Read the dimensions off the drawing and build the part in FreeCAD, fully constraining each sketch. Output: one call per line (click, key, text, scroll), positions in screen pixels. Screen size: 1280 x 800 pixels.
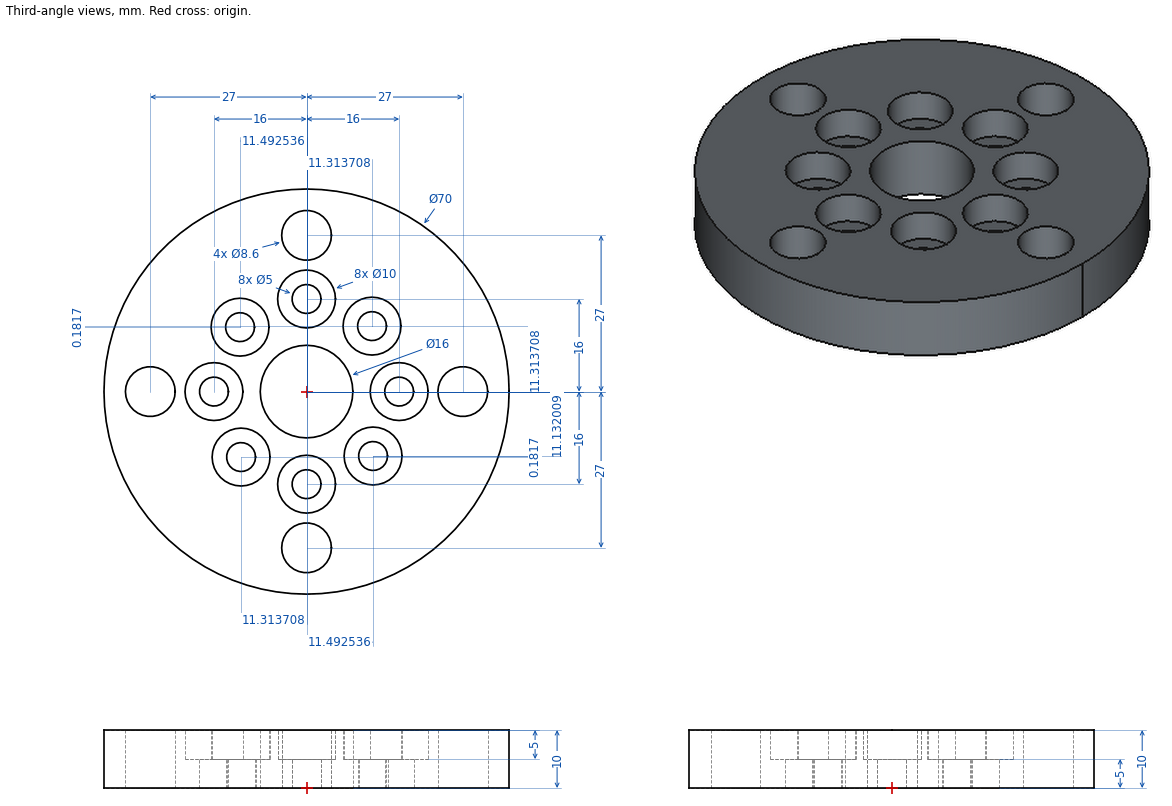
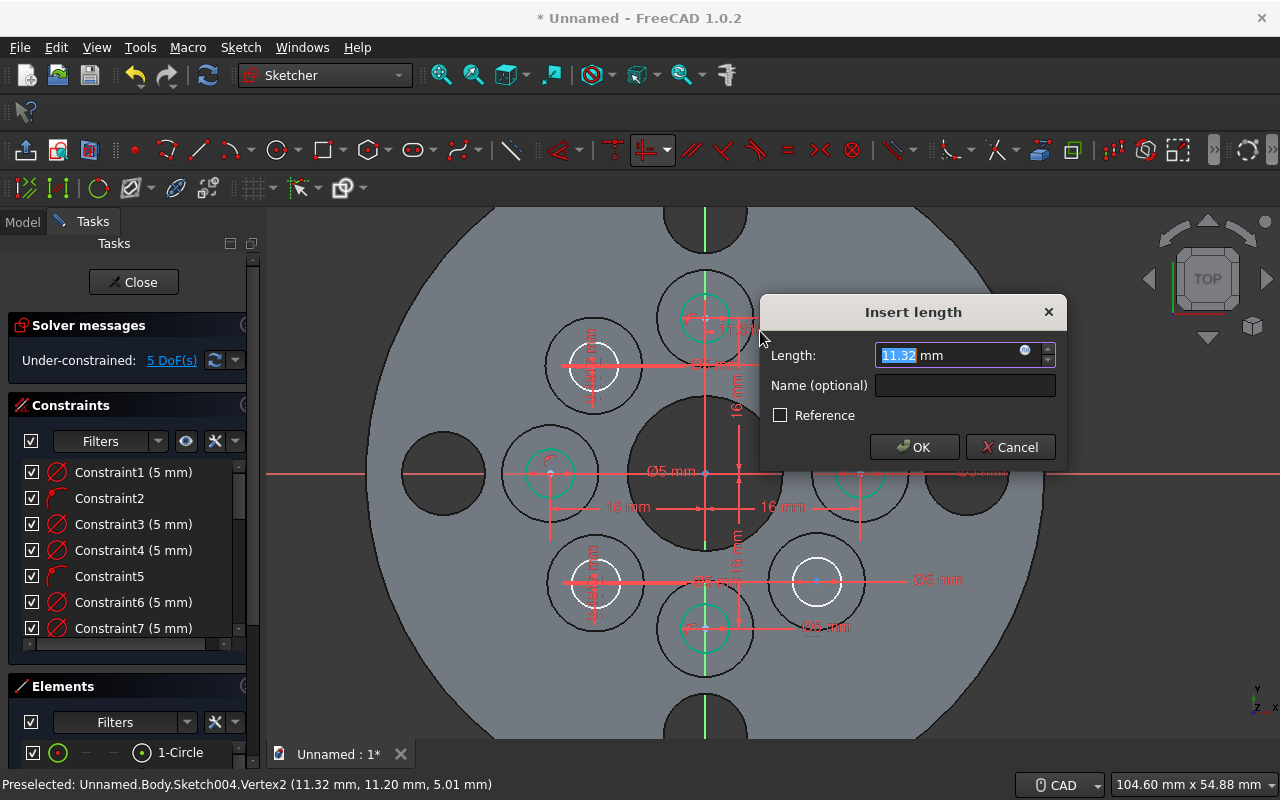
text(11.313708)
key(Return)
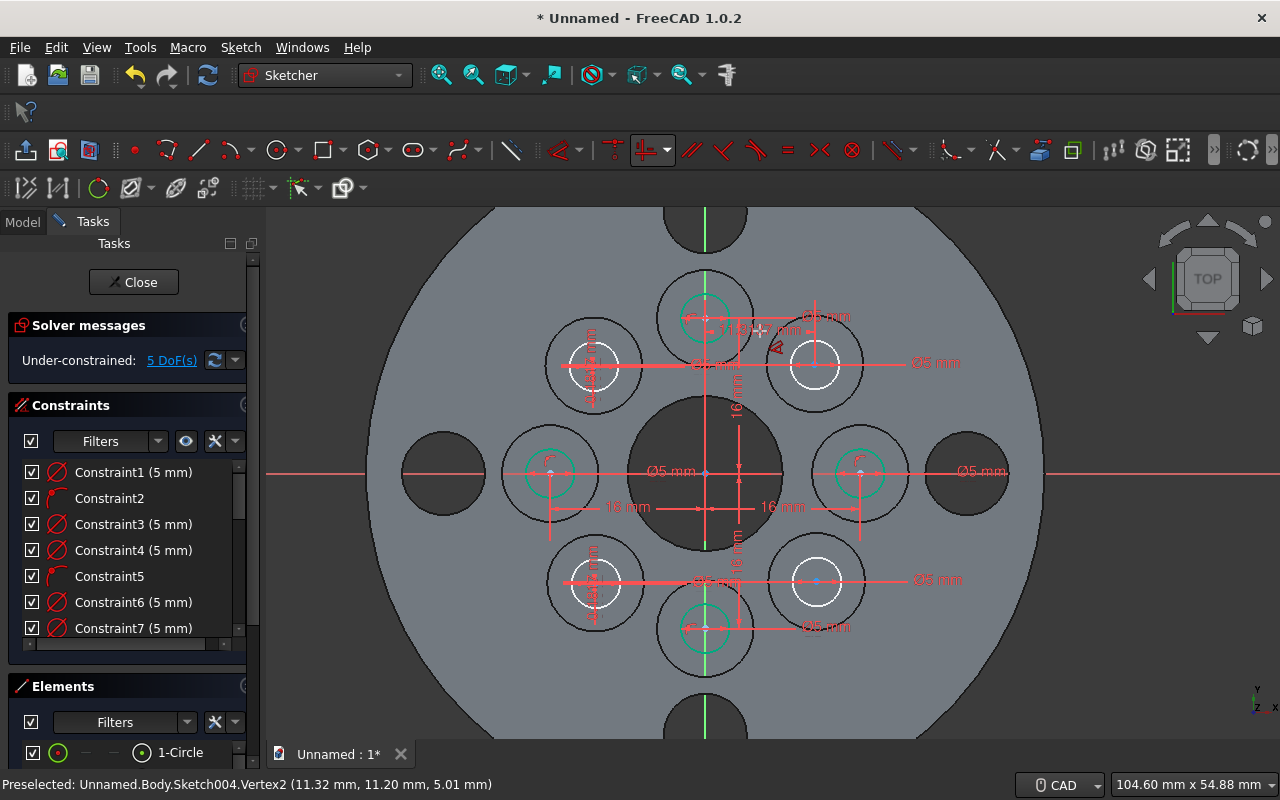
click(815, 365)
click(849, 419)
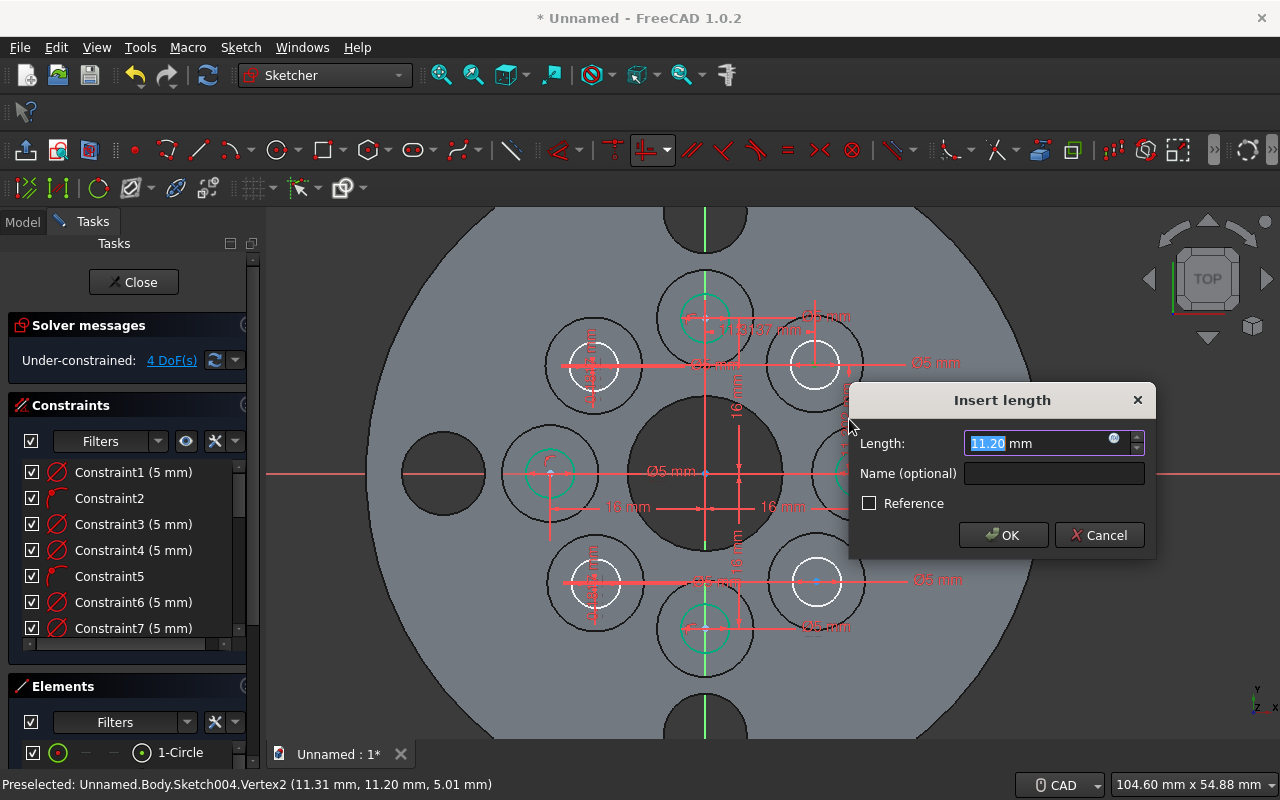
text(11.313708)
key(Return)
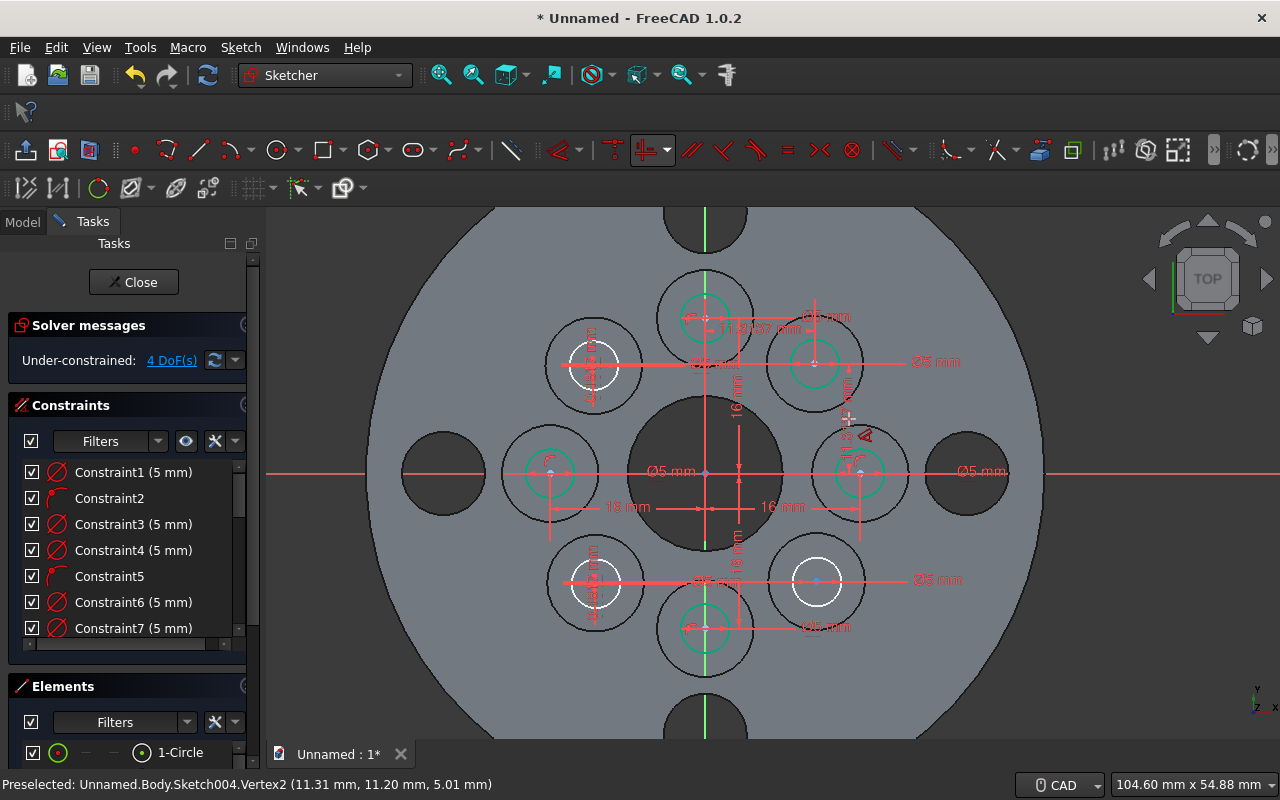
click(817, 582)
click(761, 616)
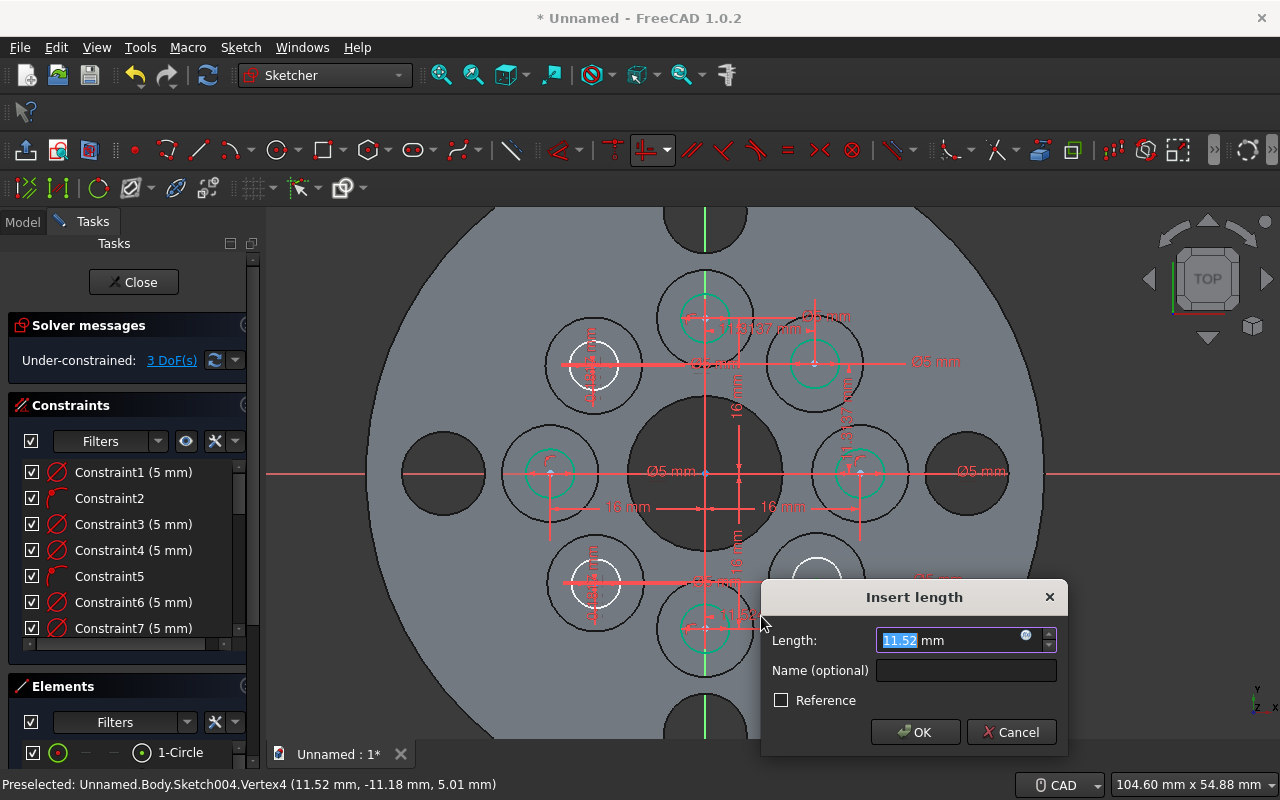
text(11.492536)
key(Return)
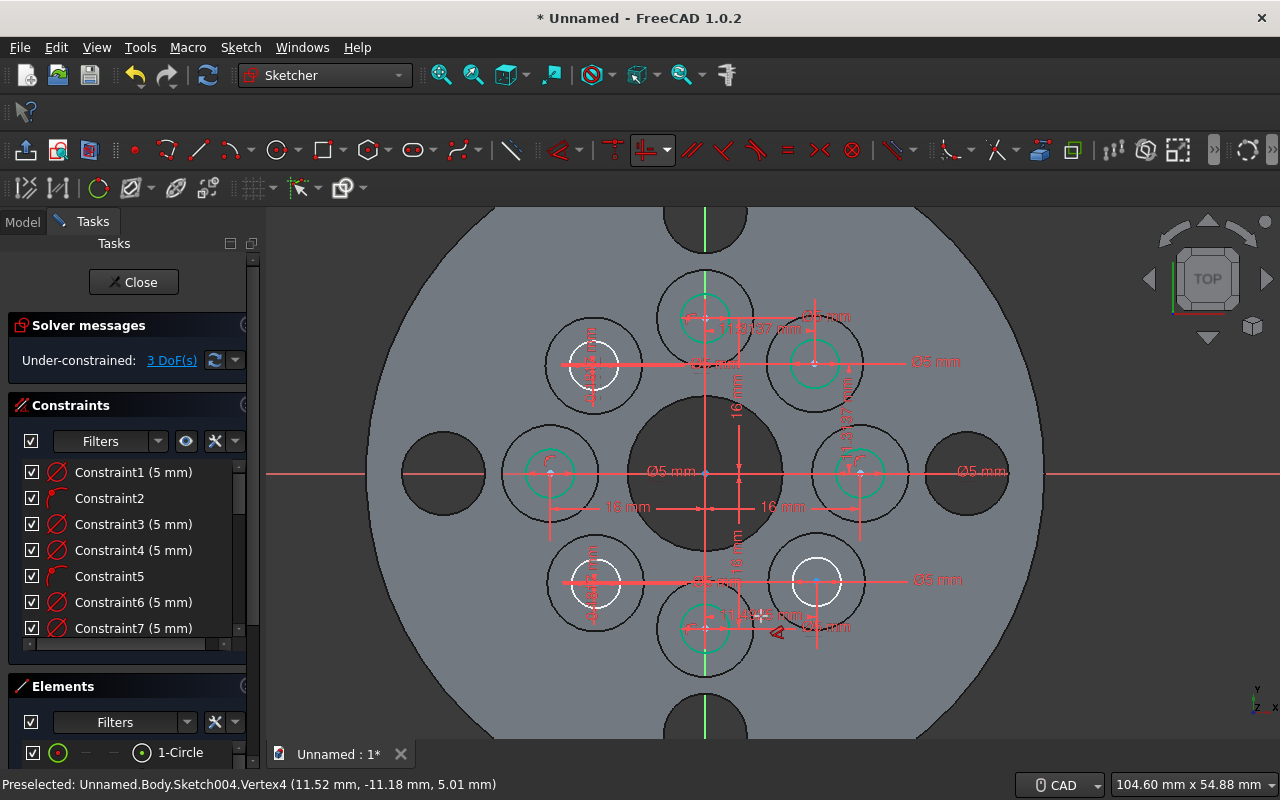
click(817, 582)
click(851, 528)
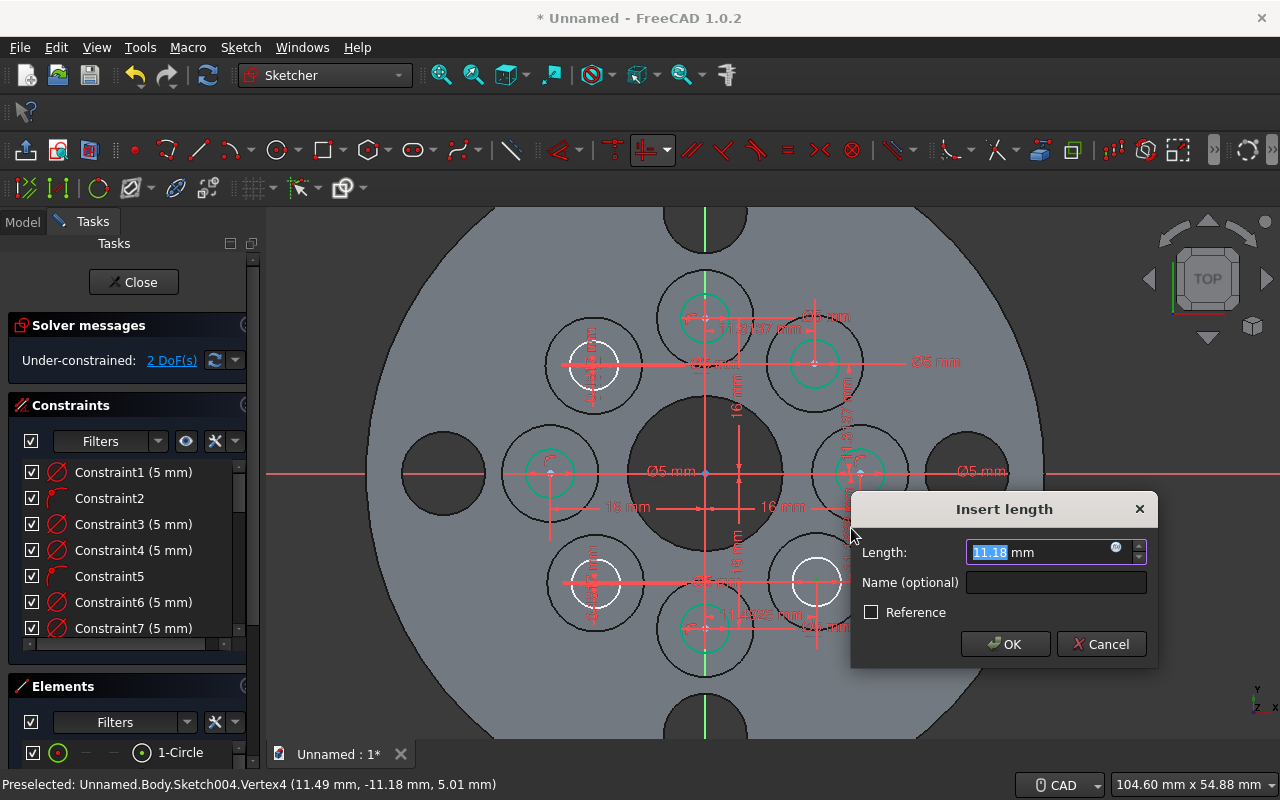
text(11.132009)
key(Return)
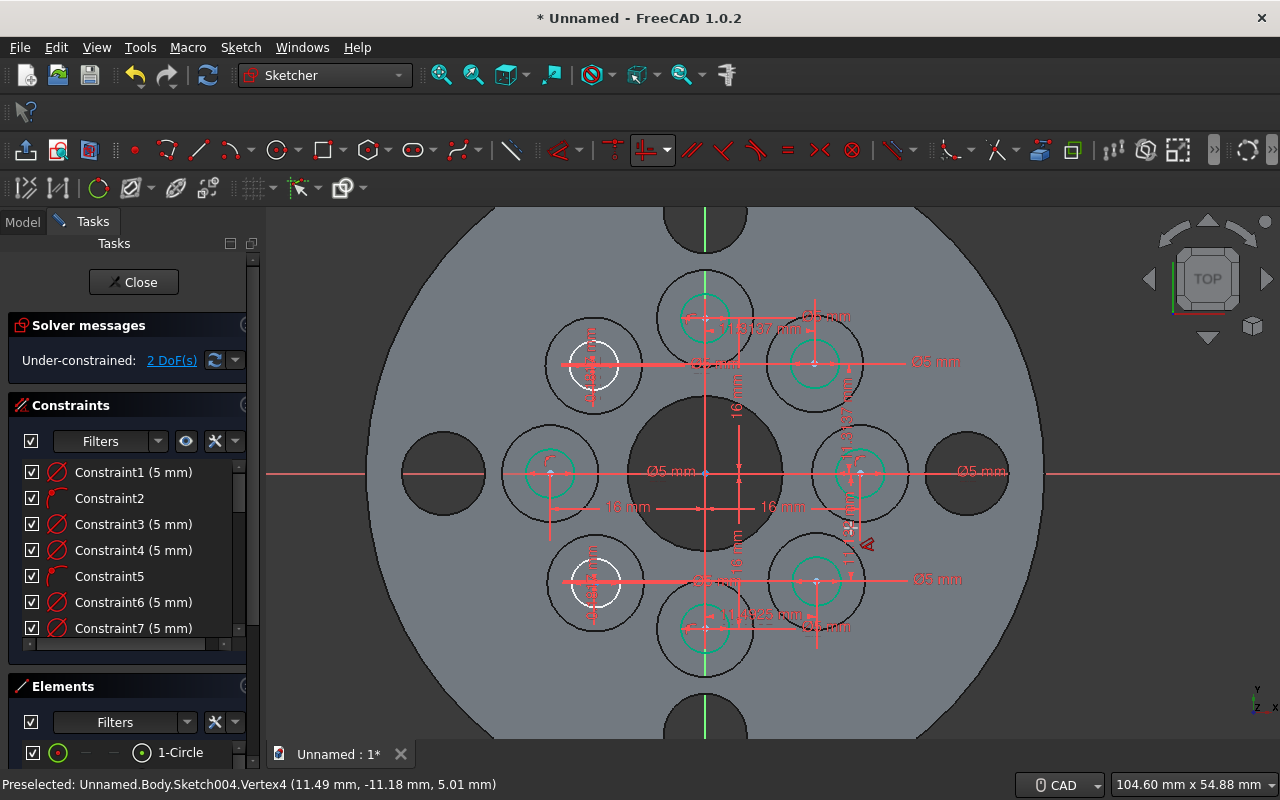
click(596, 583)
click(651, 617)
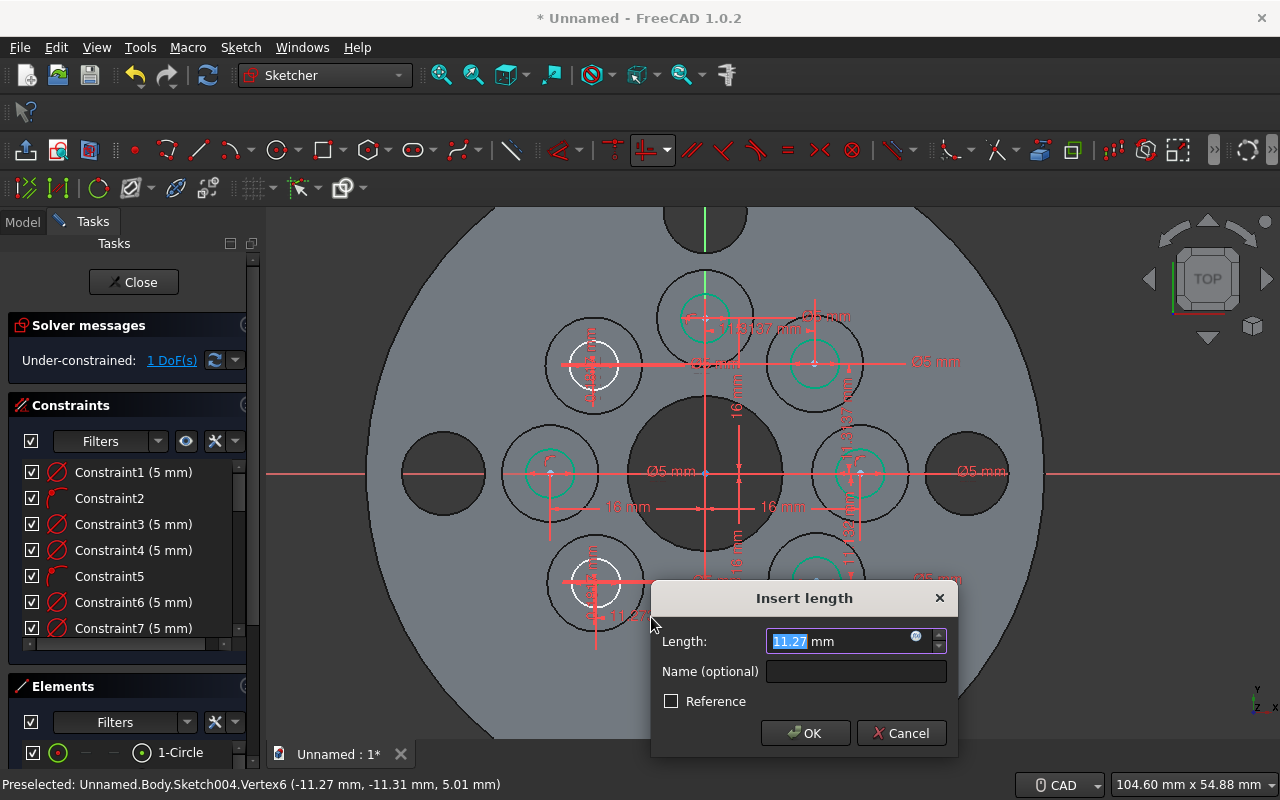
text(11.313708)
key(Return)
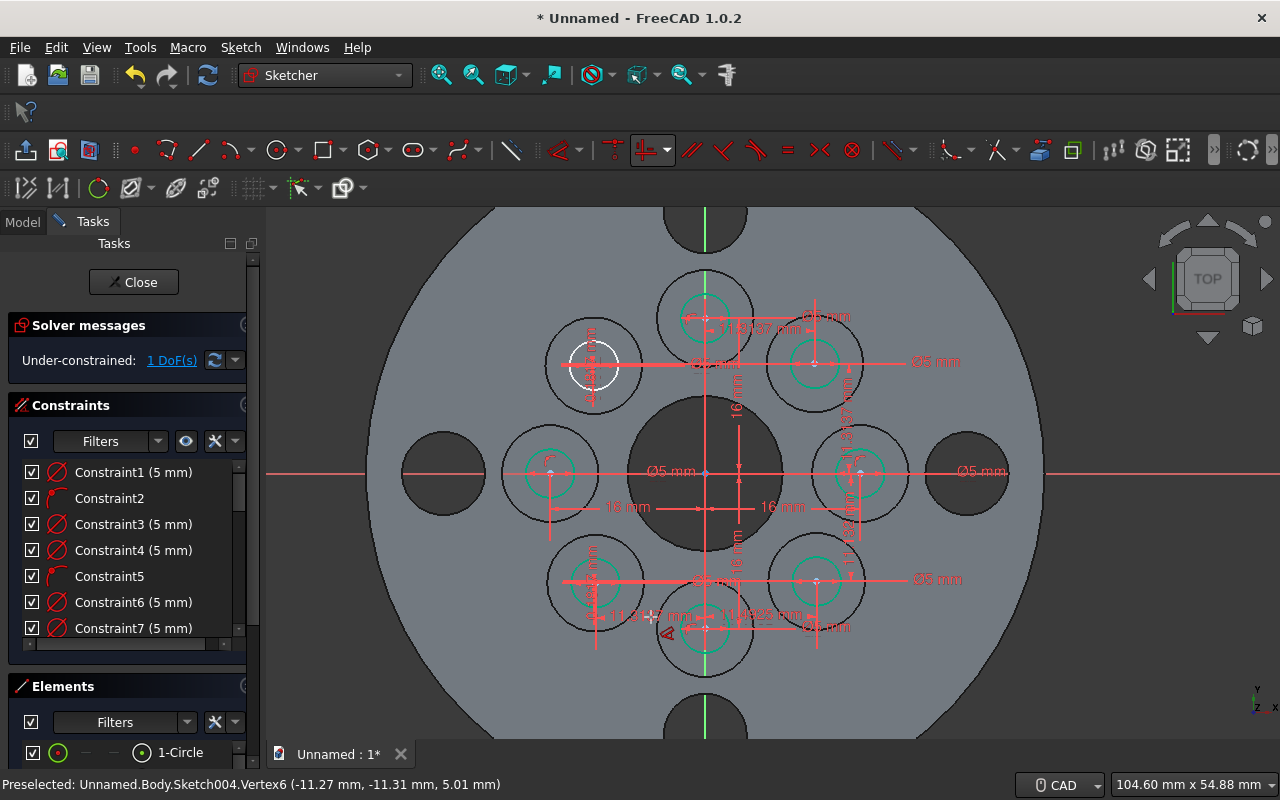
click(594, 366)
click(650, 332)